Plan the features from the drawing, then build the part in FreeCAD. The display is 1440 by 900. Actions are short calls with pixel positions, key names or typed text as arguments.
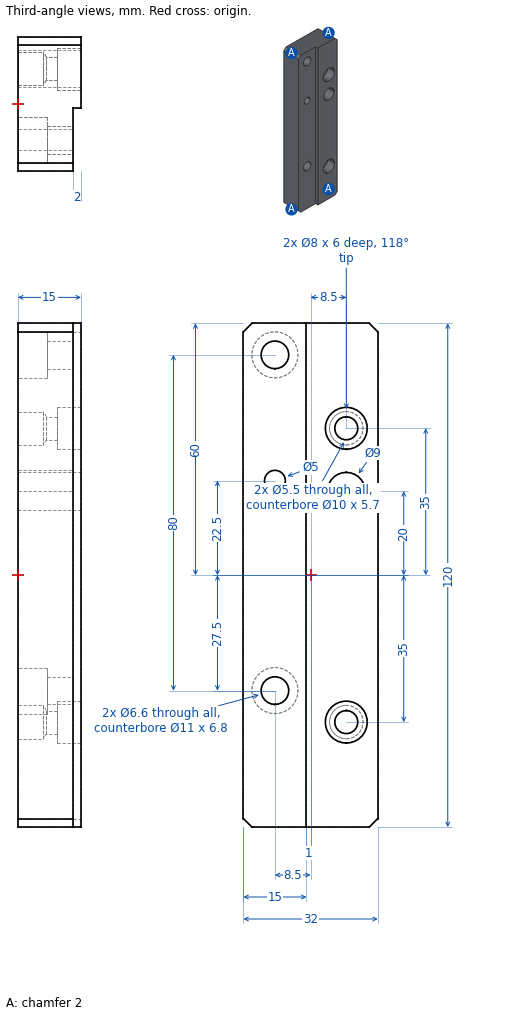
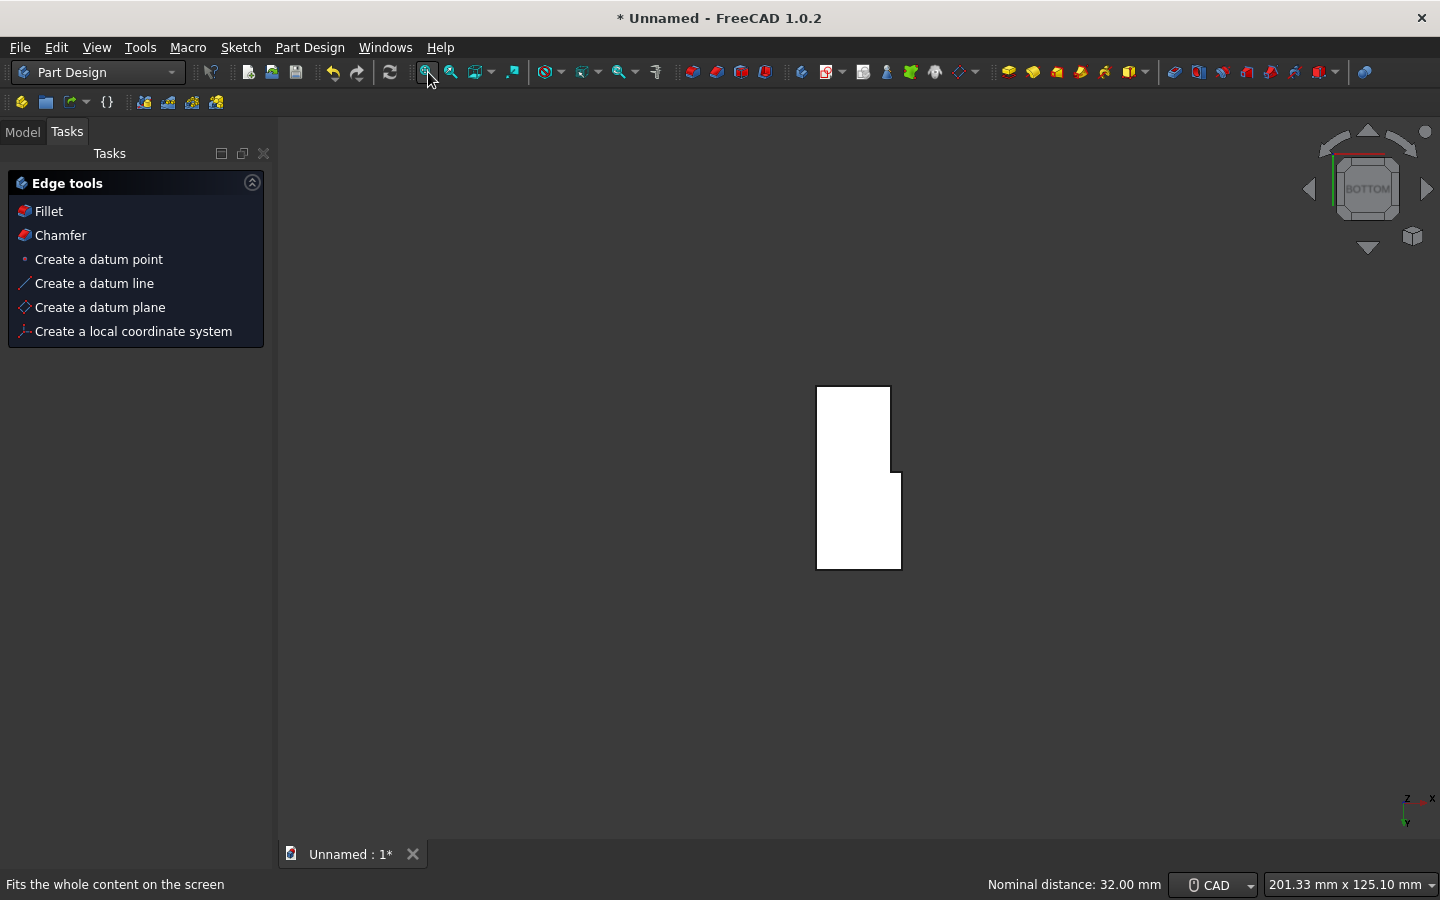
click(853, 385, ctrl)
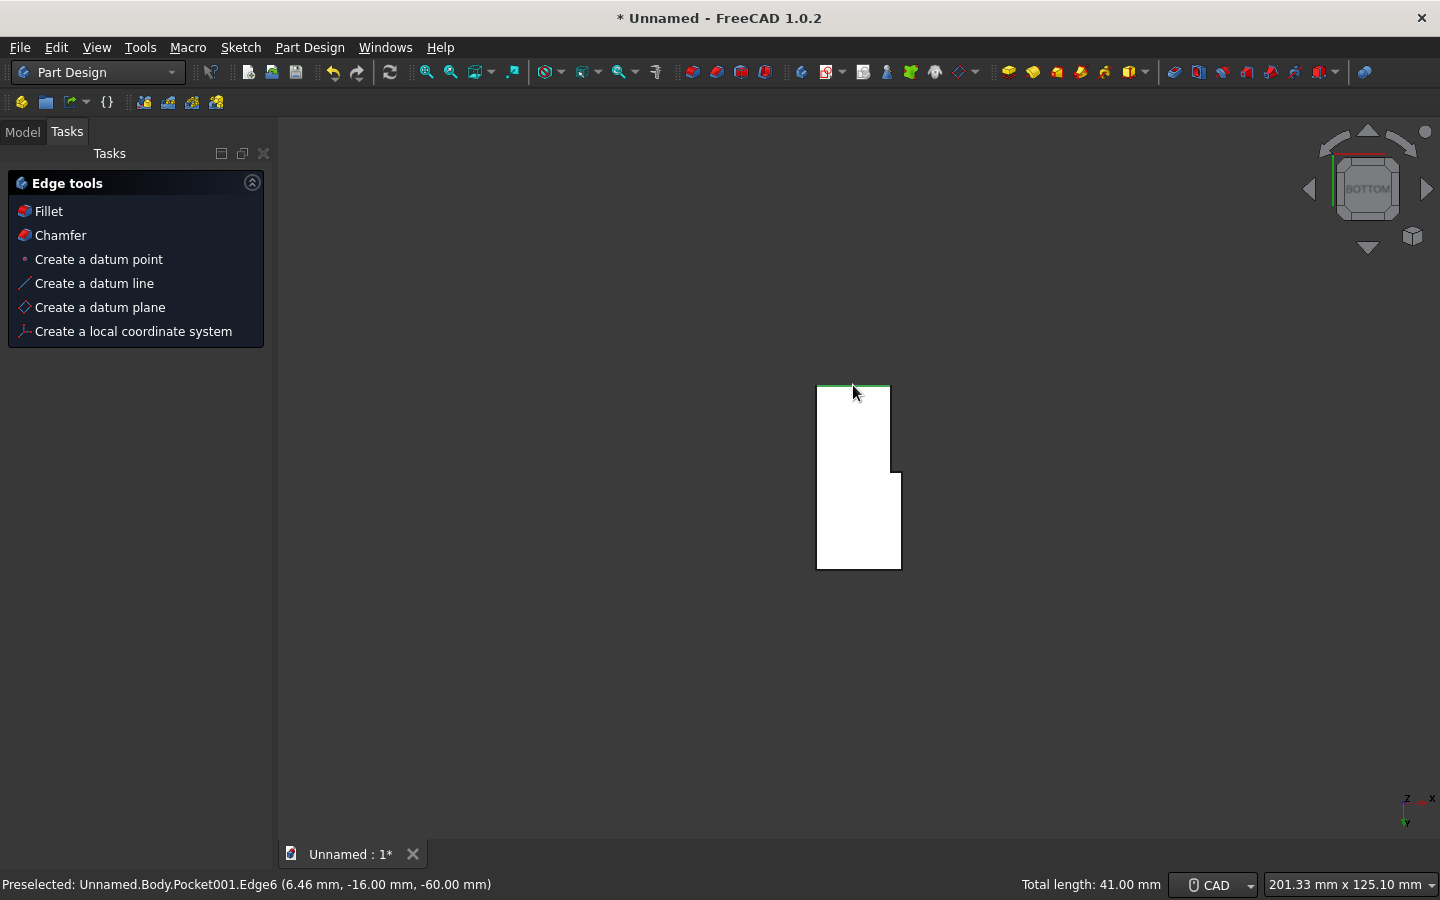
click(859, 569, ctrl)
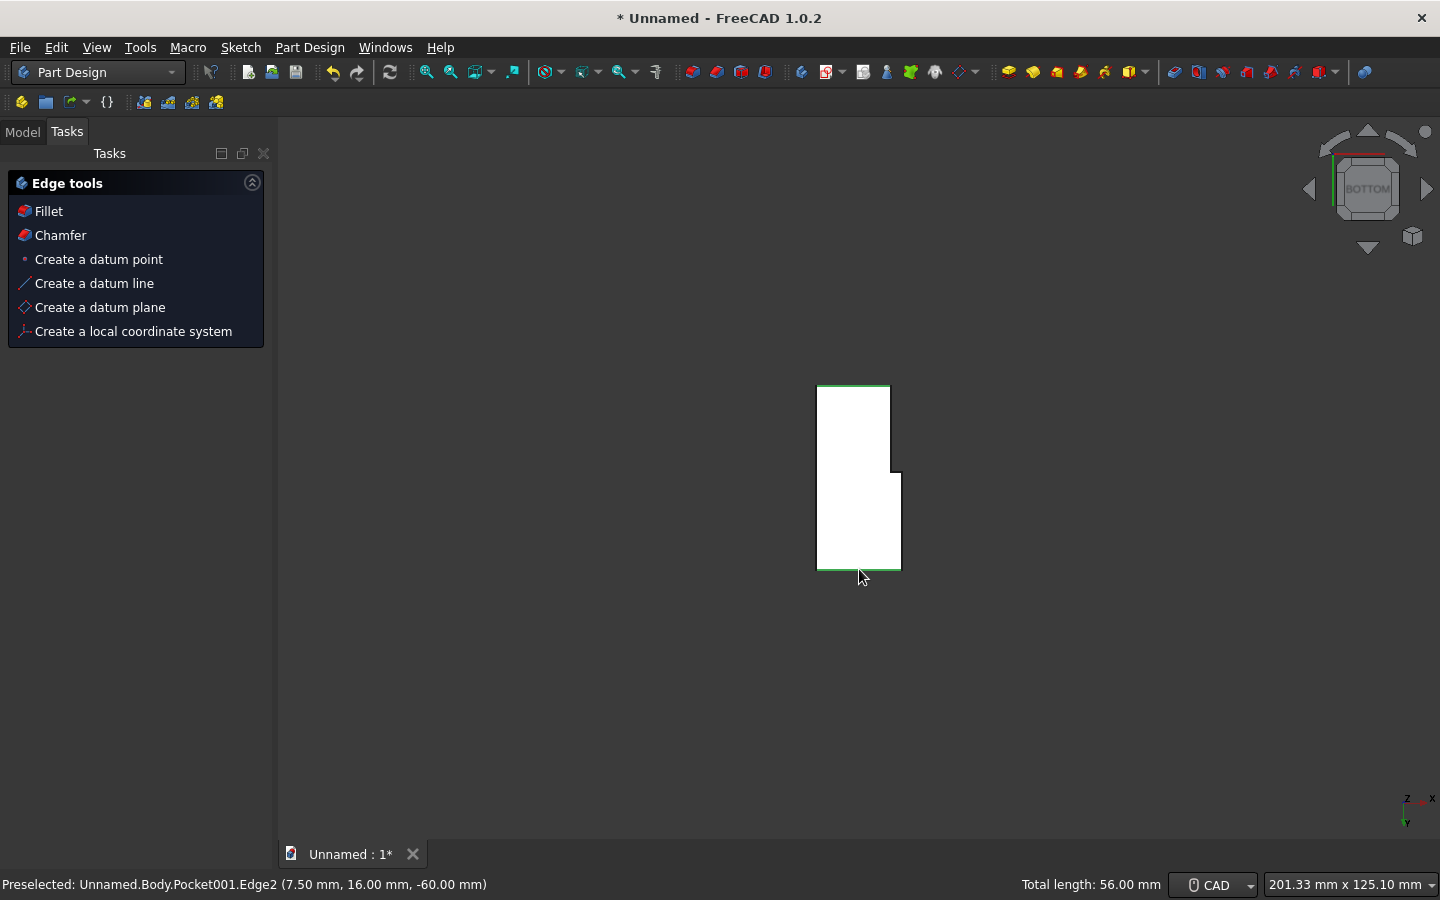
click(718, 72)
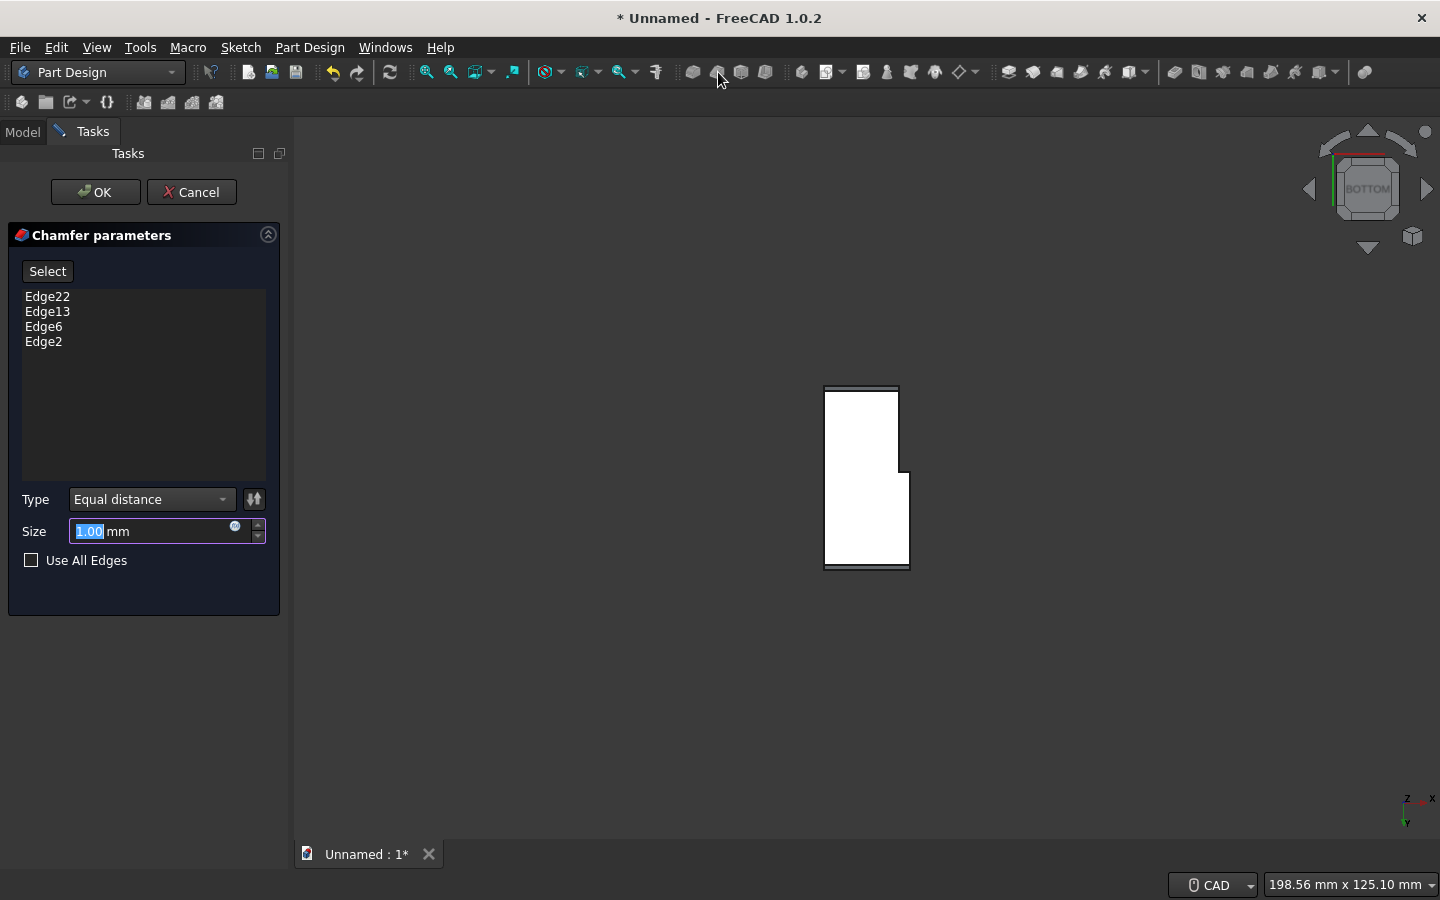
text(2)
key(Tab)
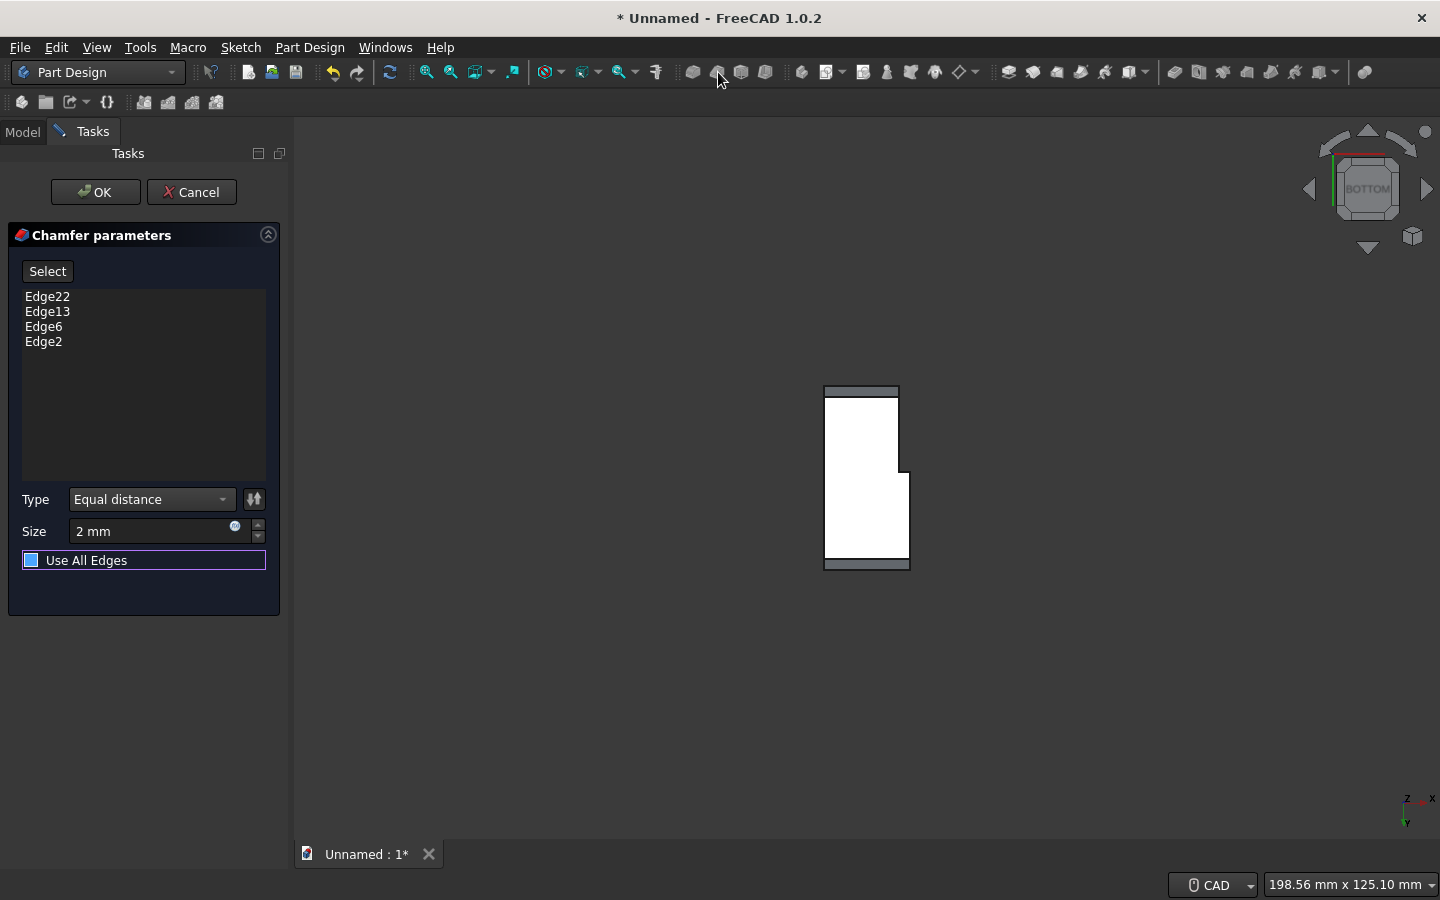
click(96, 192)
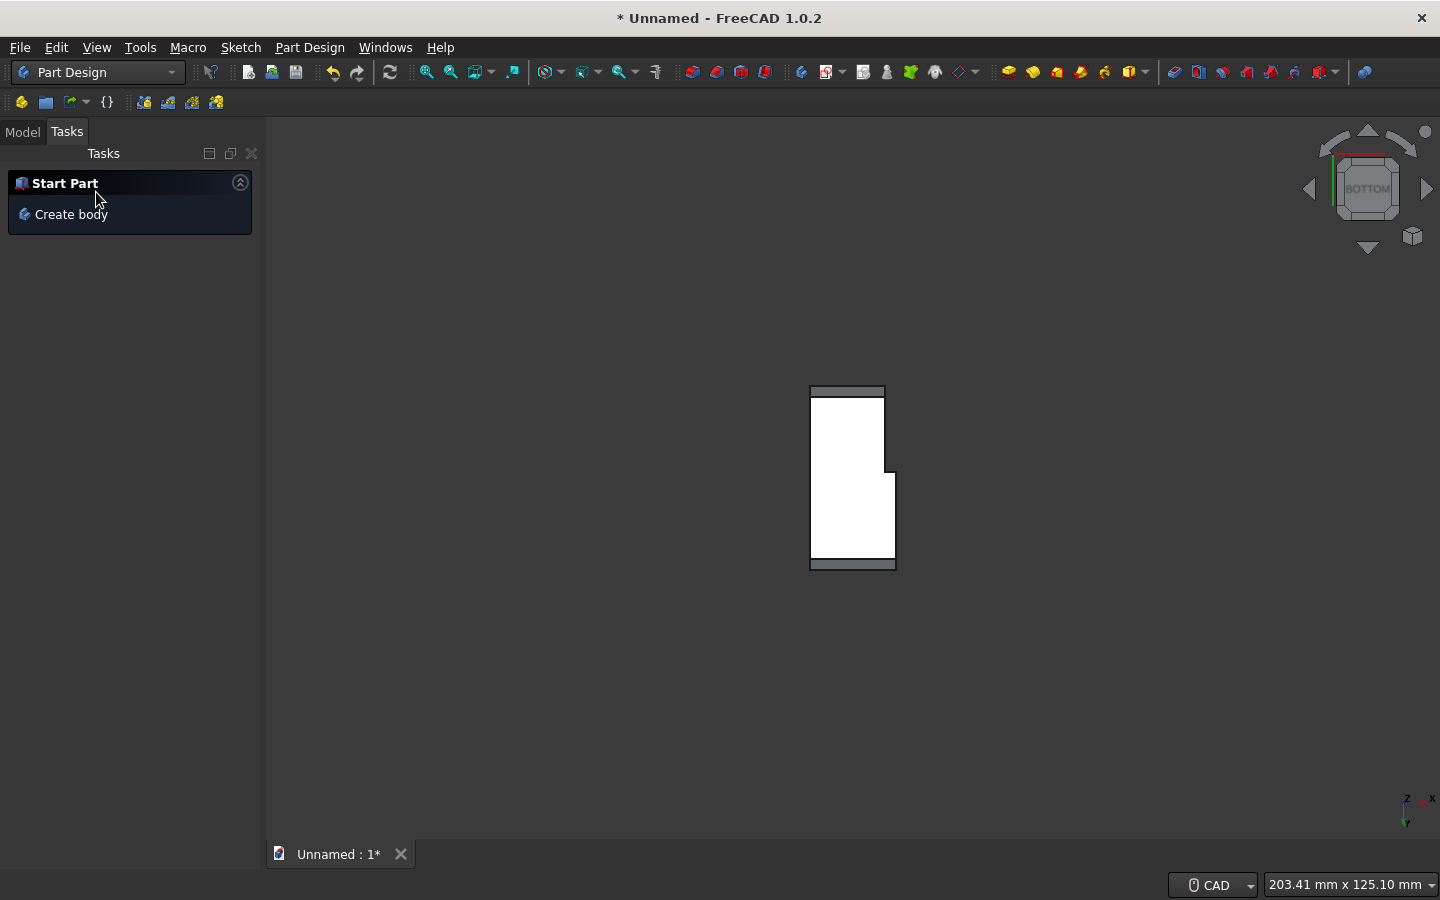
click(428, 72)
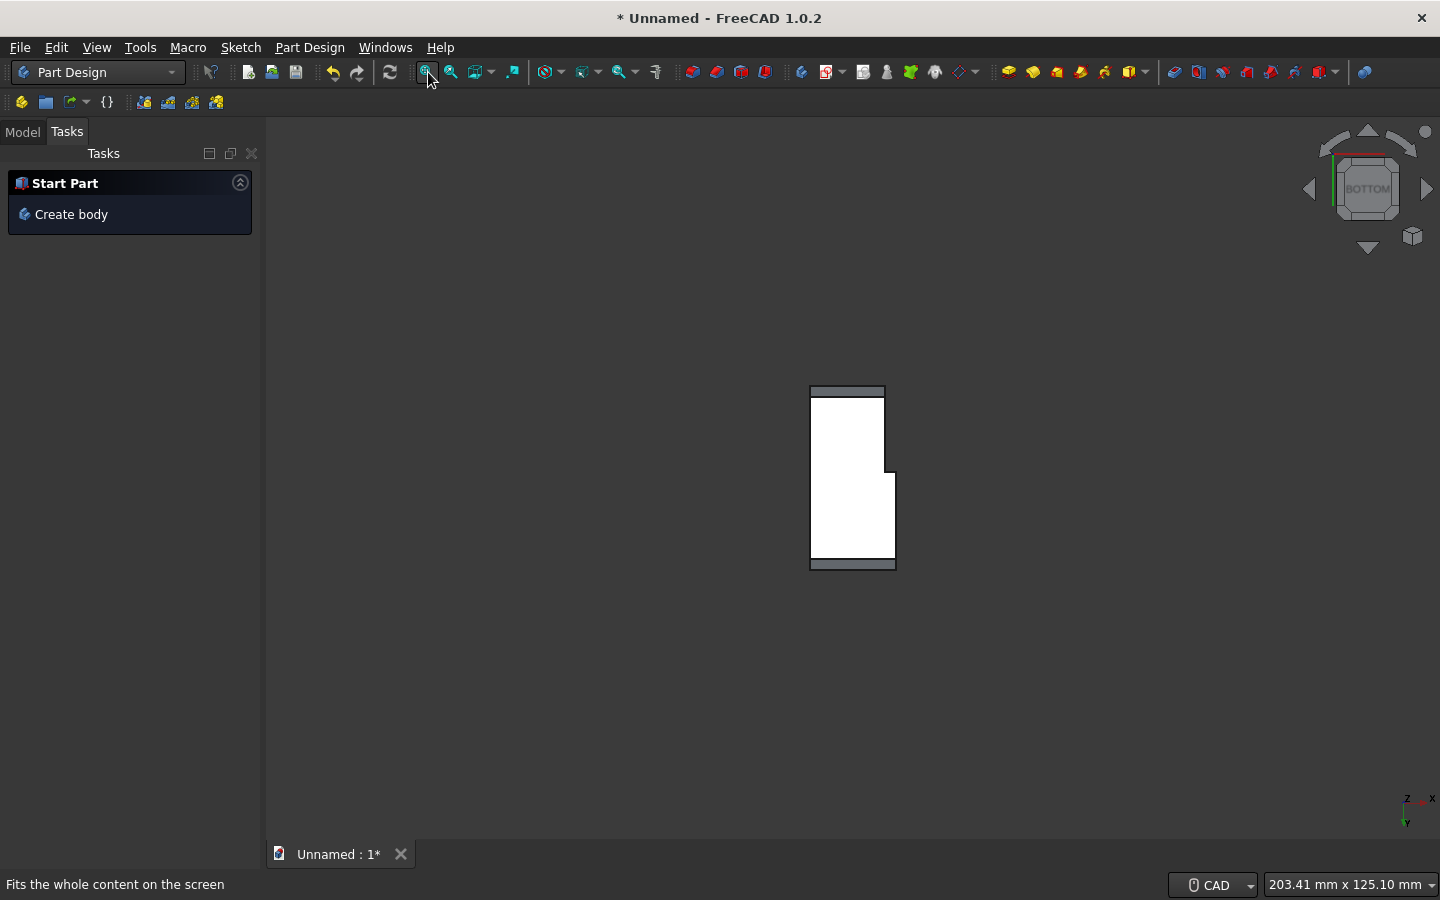
key(0)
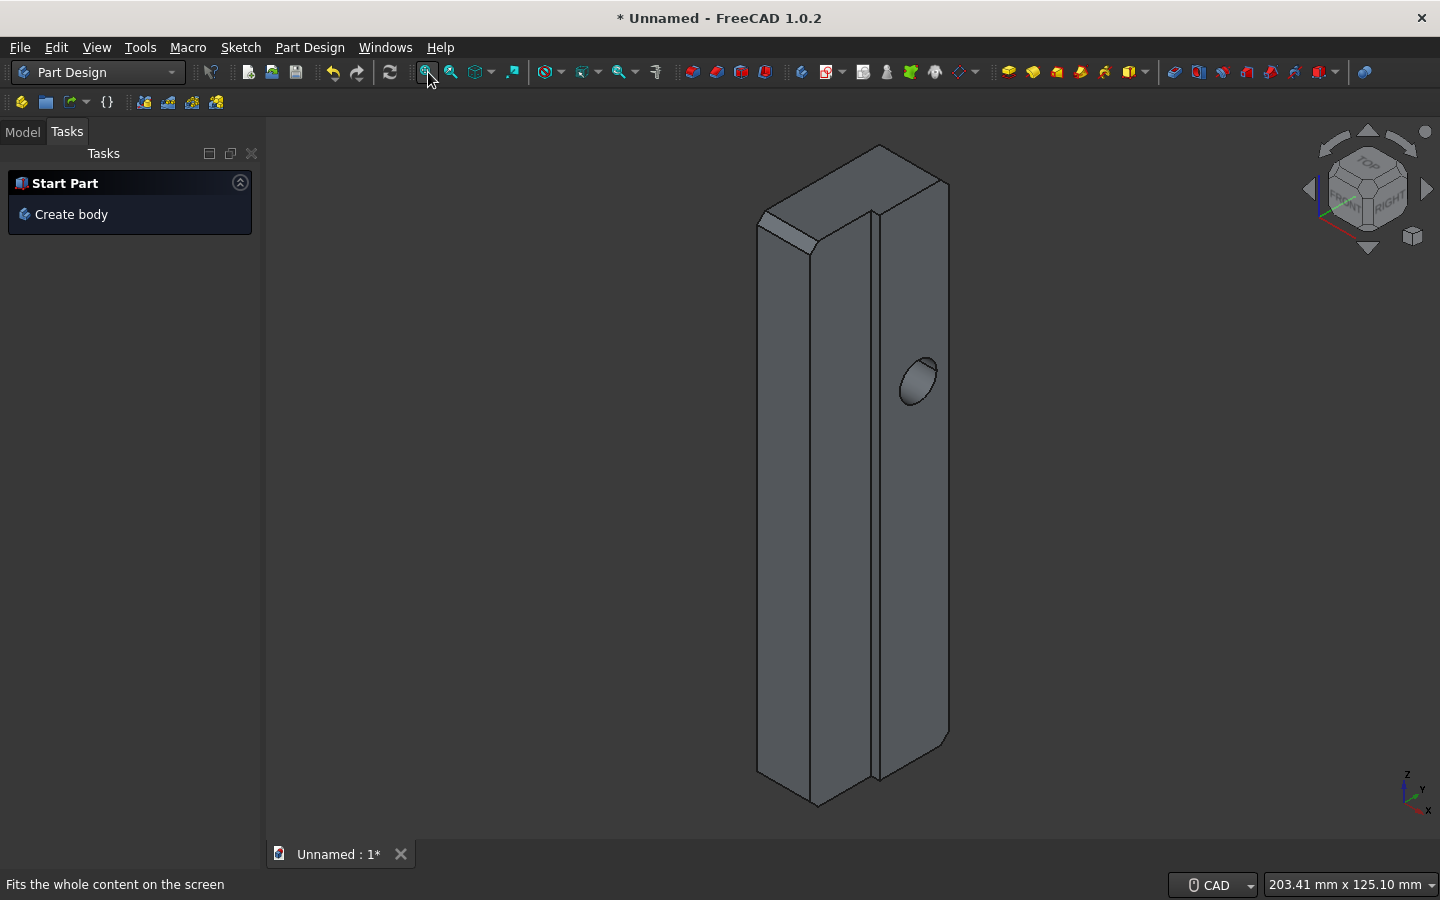
click(914, 558)